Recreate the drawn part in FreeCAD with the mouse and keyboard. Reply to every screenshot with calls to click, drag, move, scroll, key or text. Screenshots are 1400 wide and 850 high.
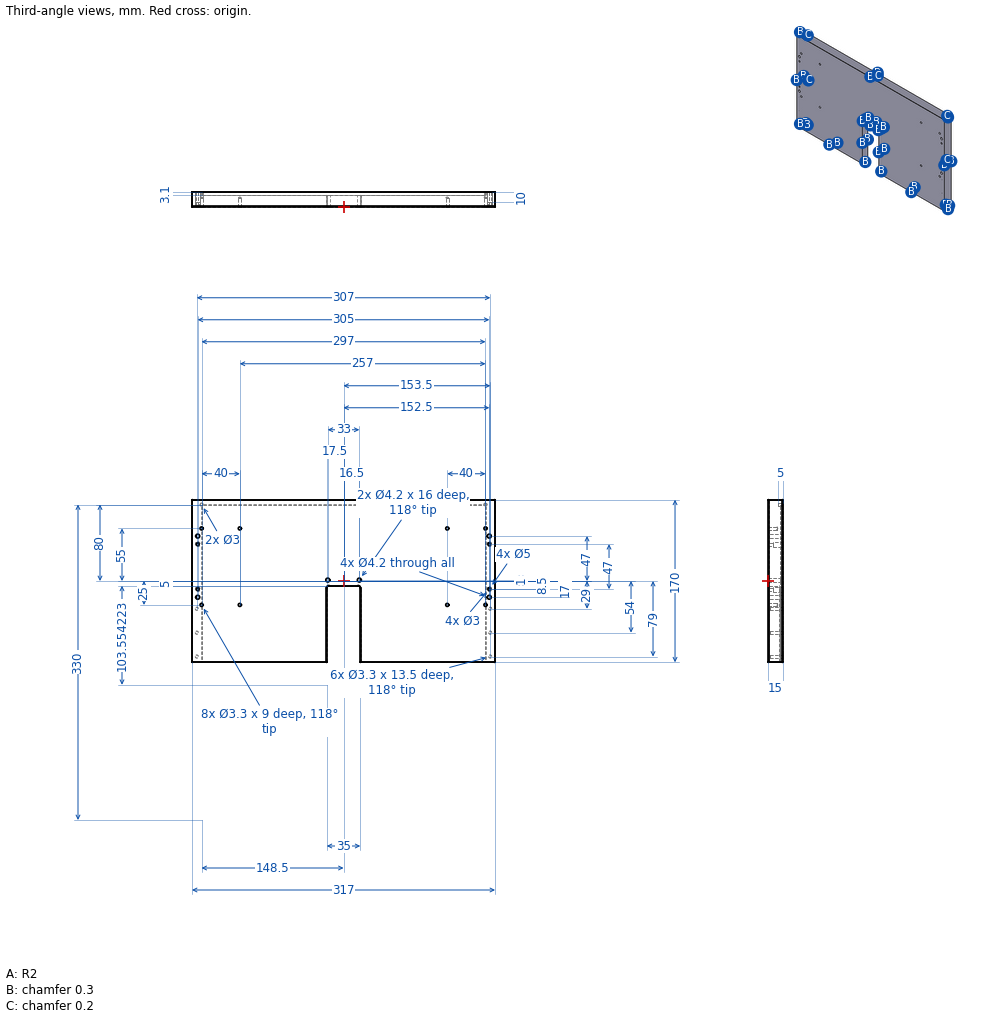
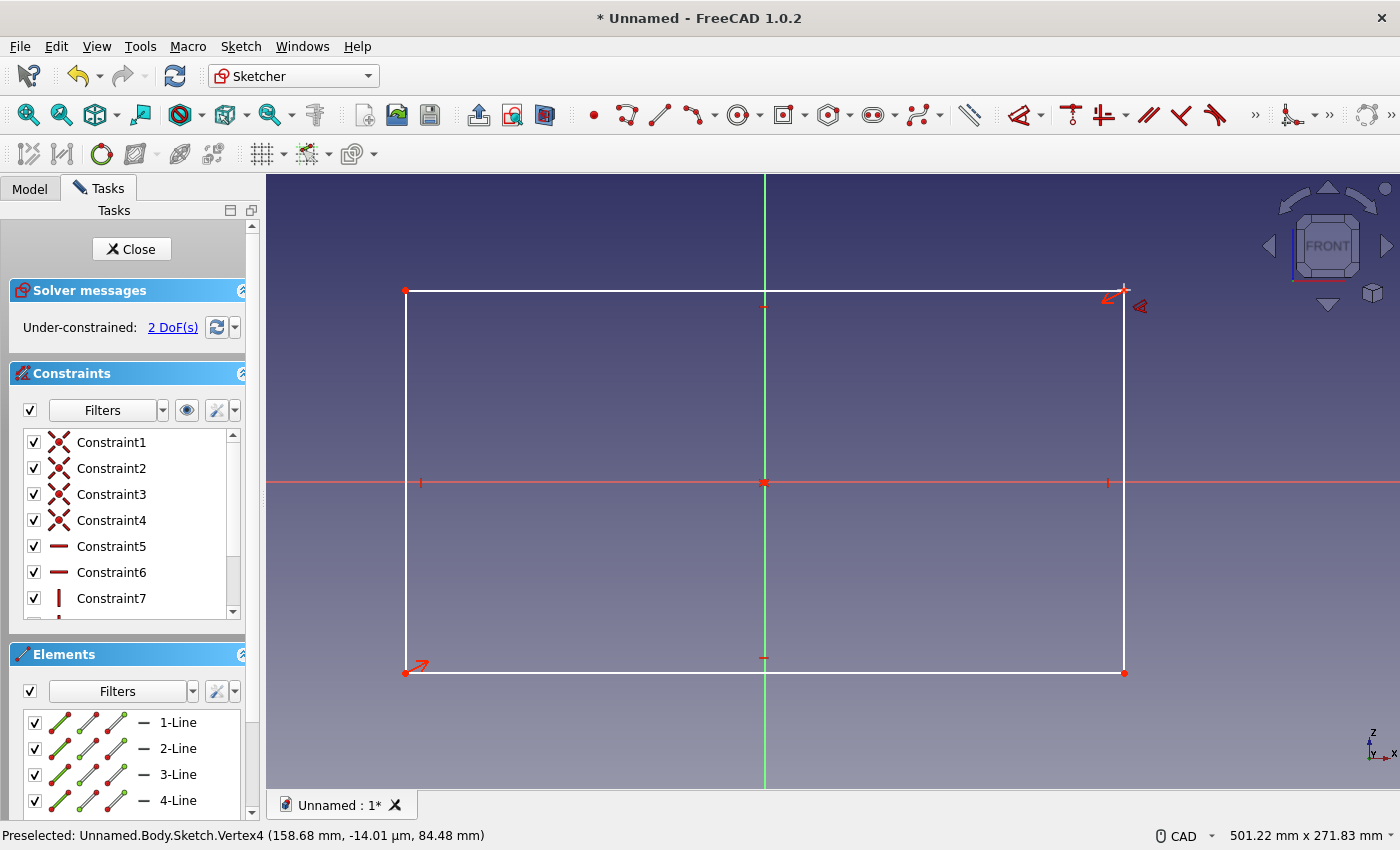
click(621, 673)
click(600, 707)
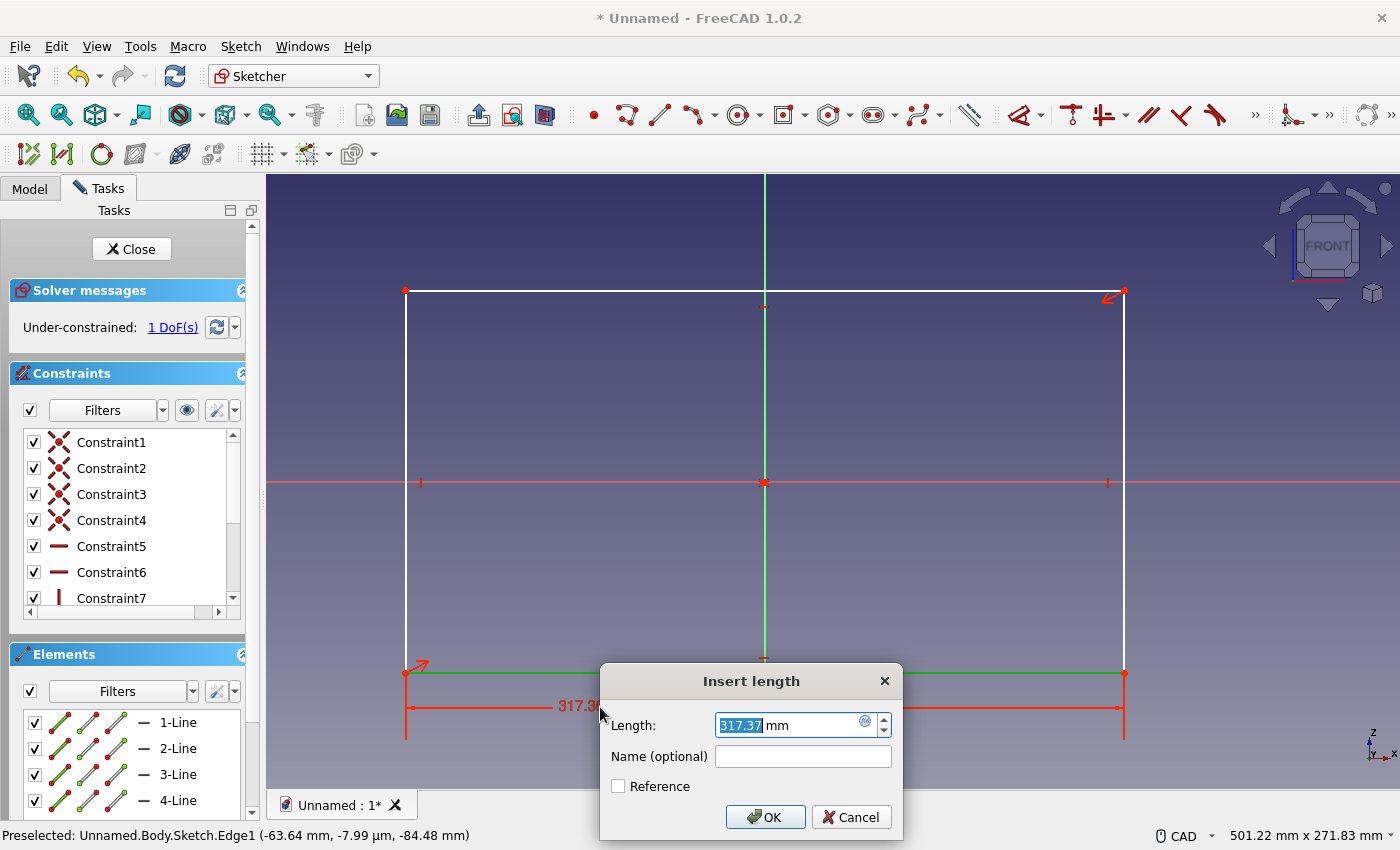
text(317)
key(Return)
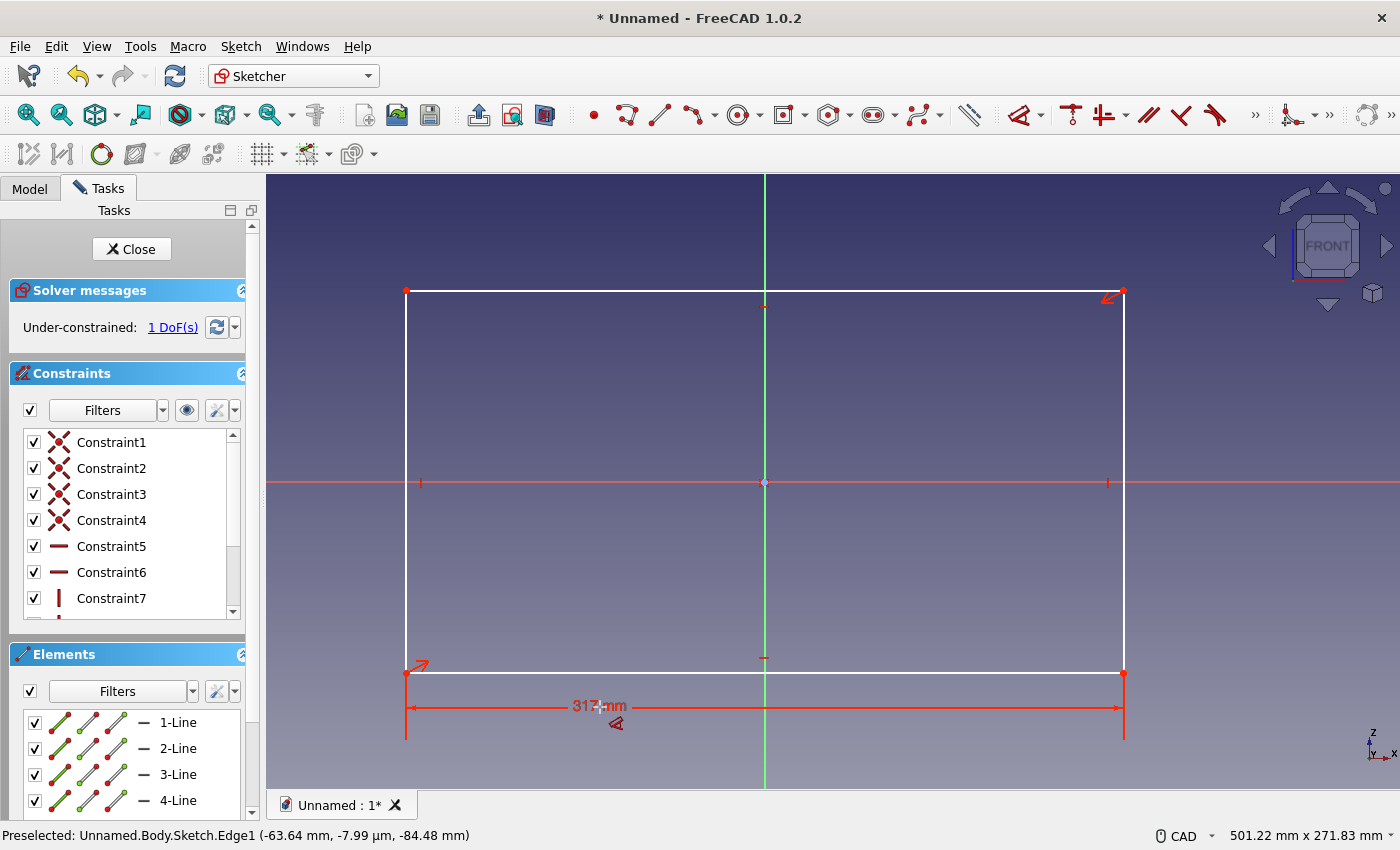
click(1124, 559)
click(1158, 394)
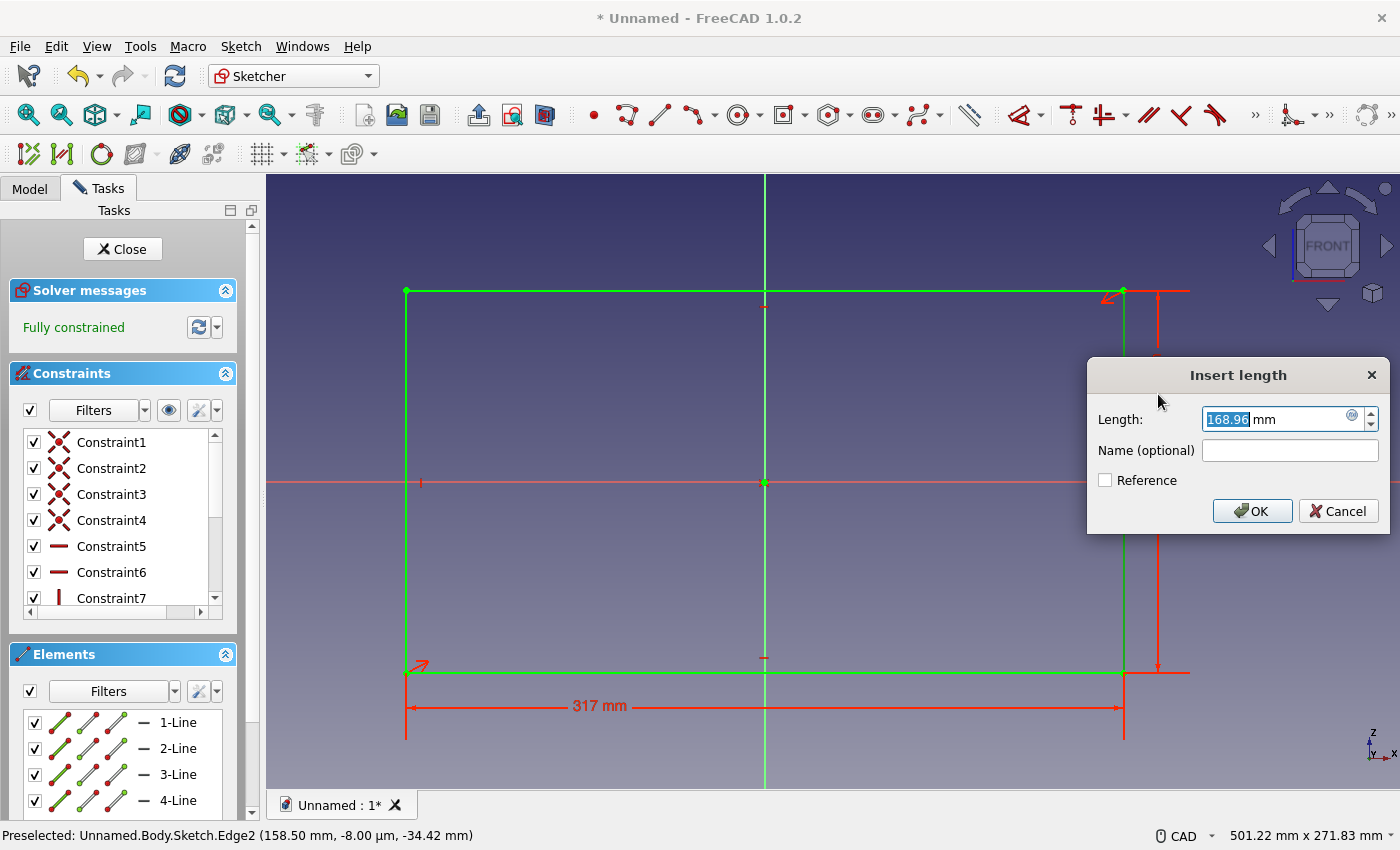
text(170)
key(Return)
key(Escape)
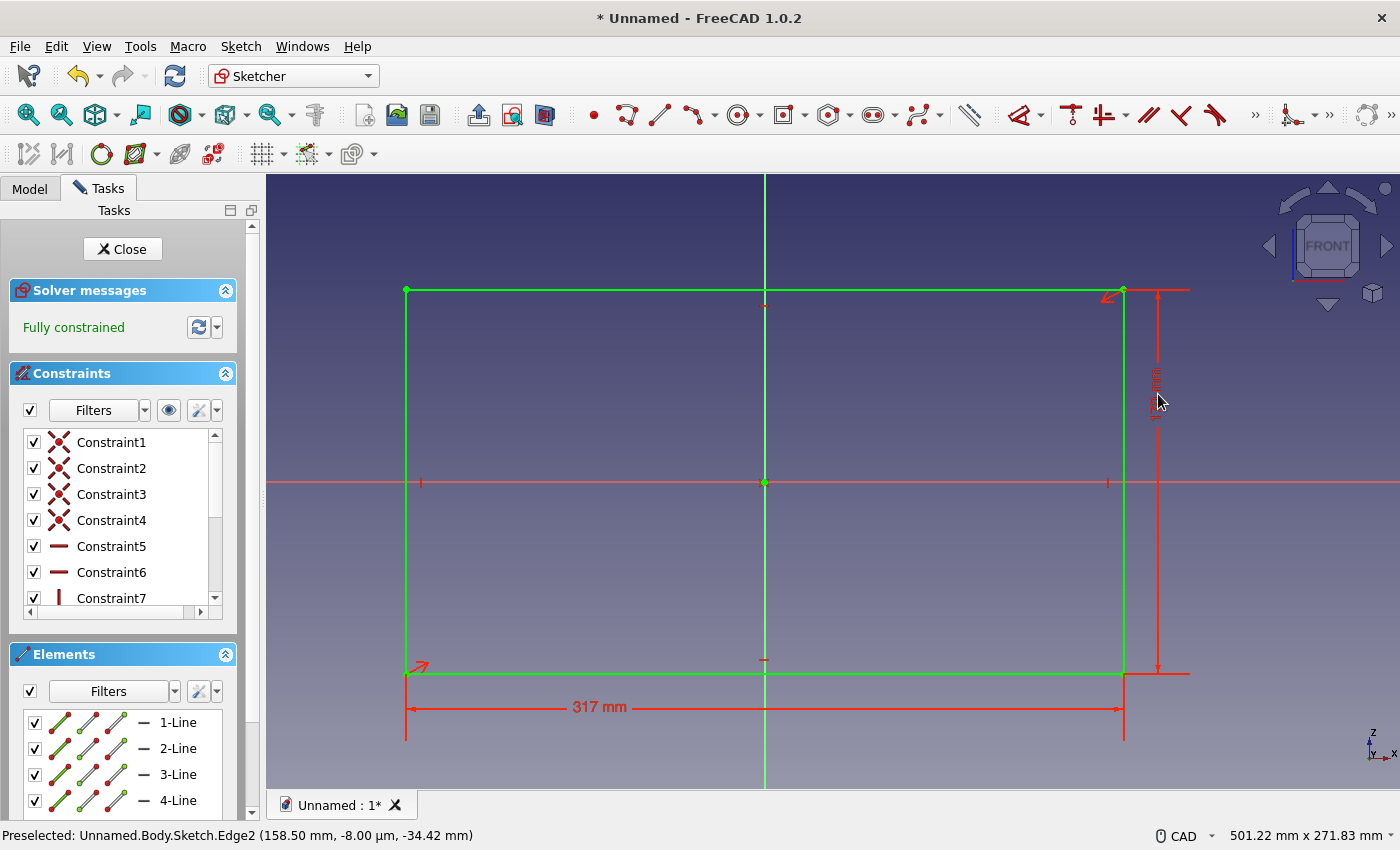
click(123, 249)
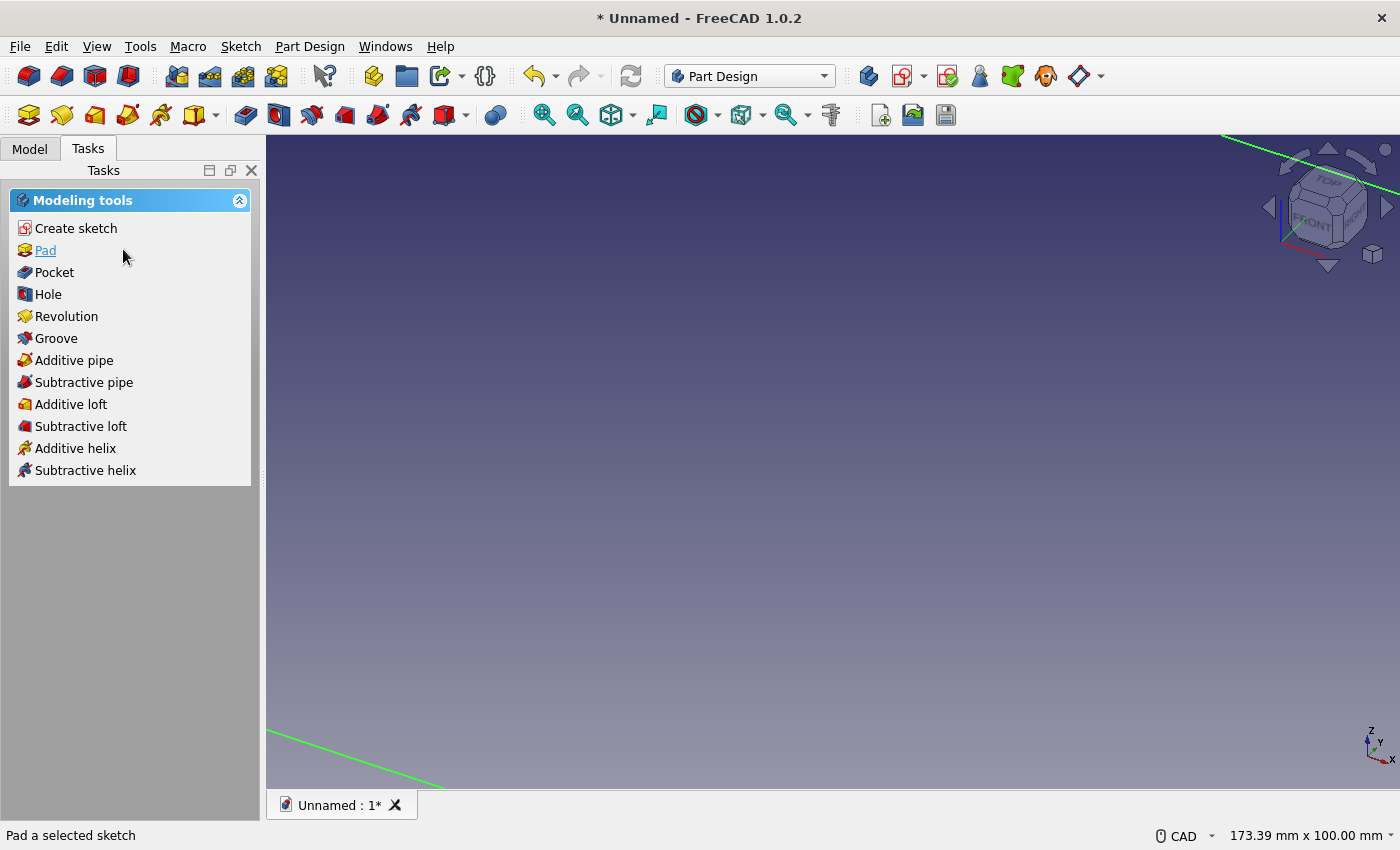
click(29, 116)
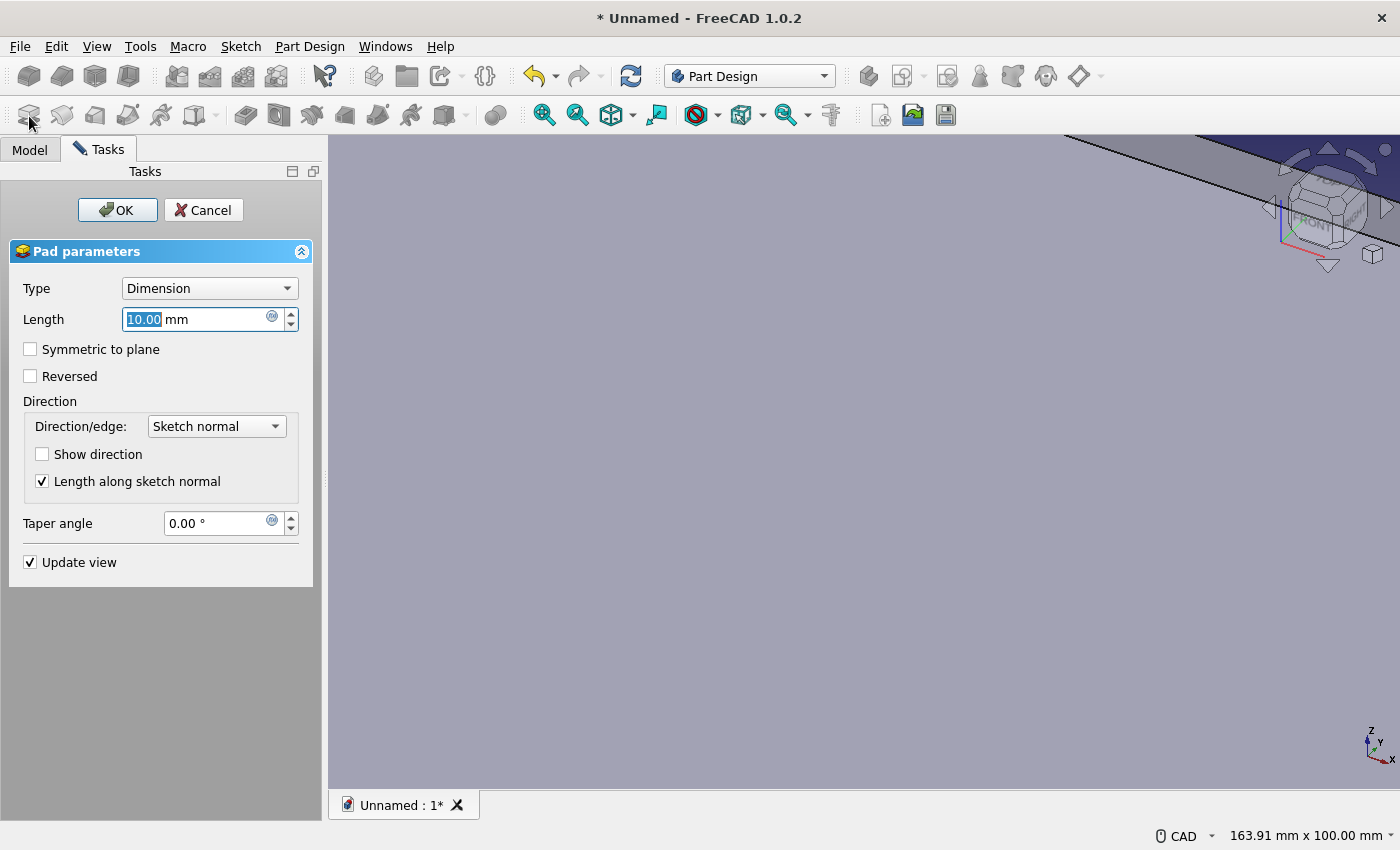
text(15)
key(Tab)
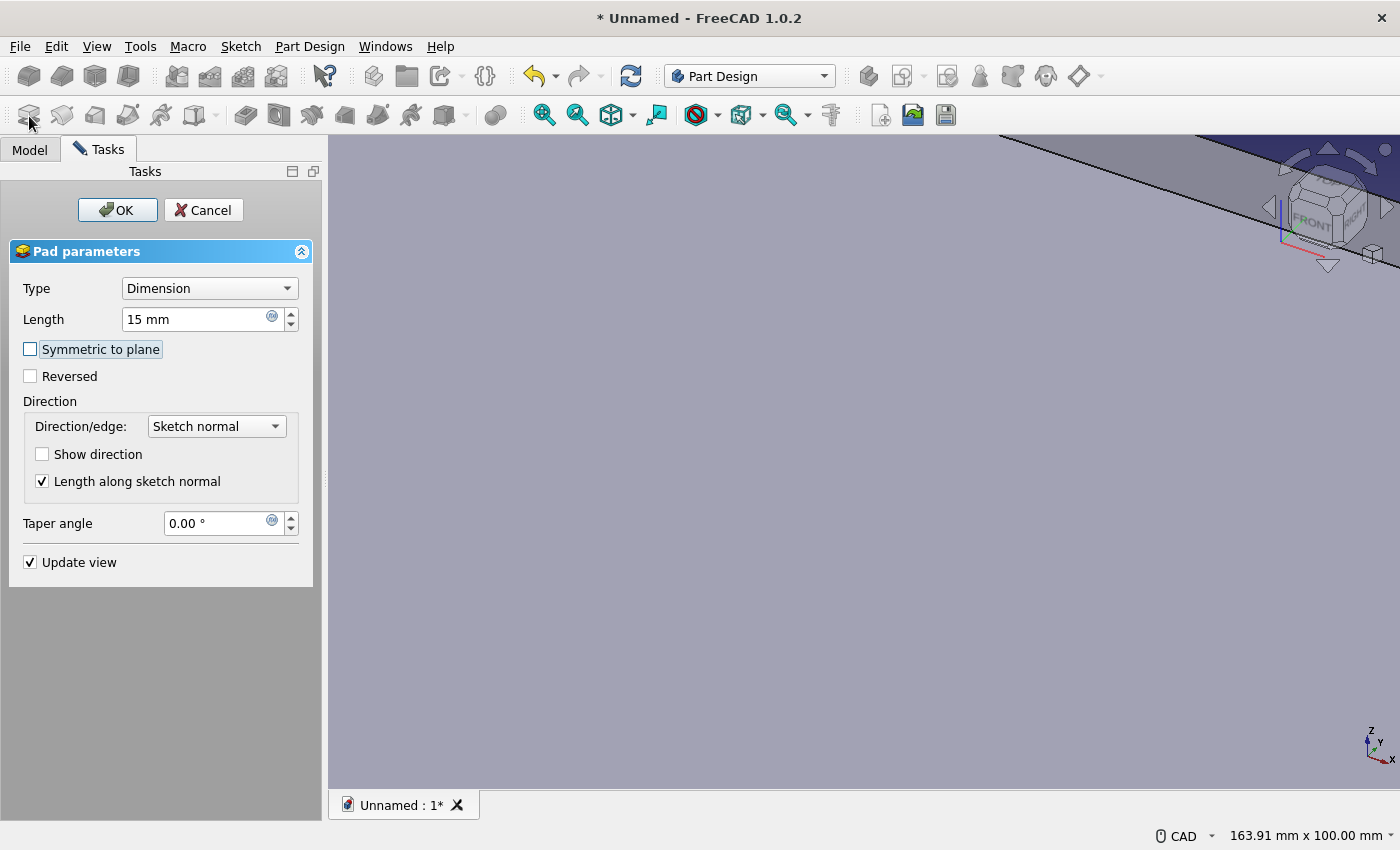
click(31, 376)